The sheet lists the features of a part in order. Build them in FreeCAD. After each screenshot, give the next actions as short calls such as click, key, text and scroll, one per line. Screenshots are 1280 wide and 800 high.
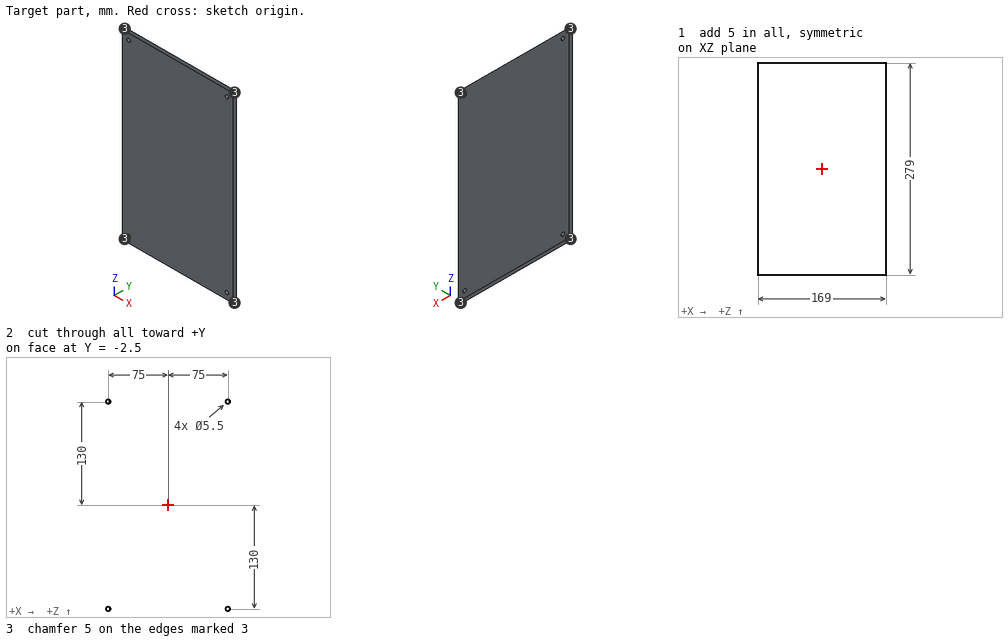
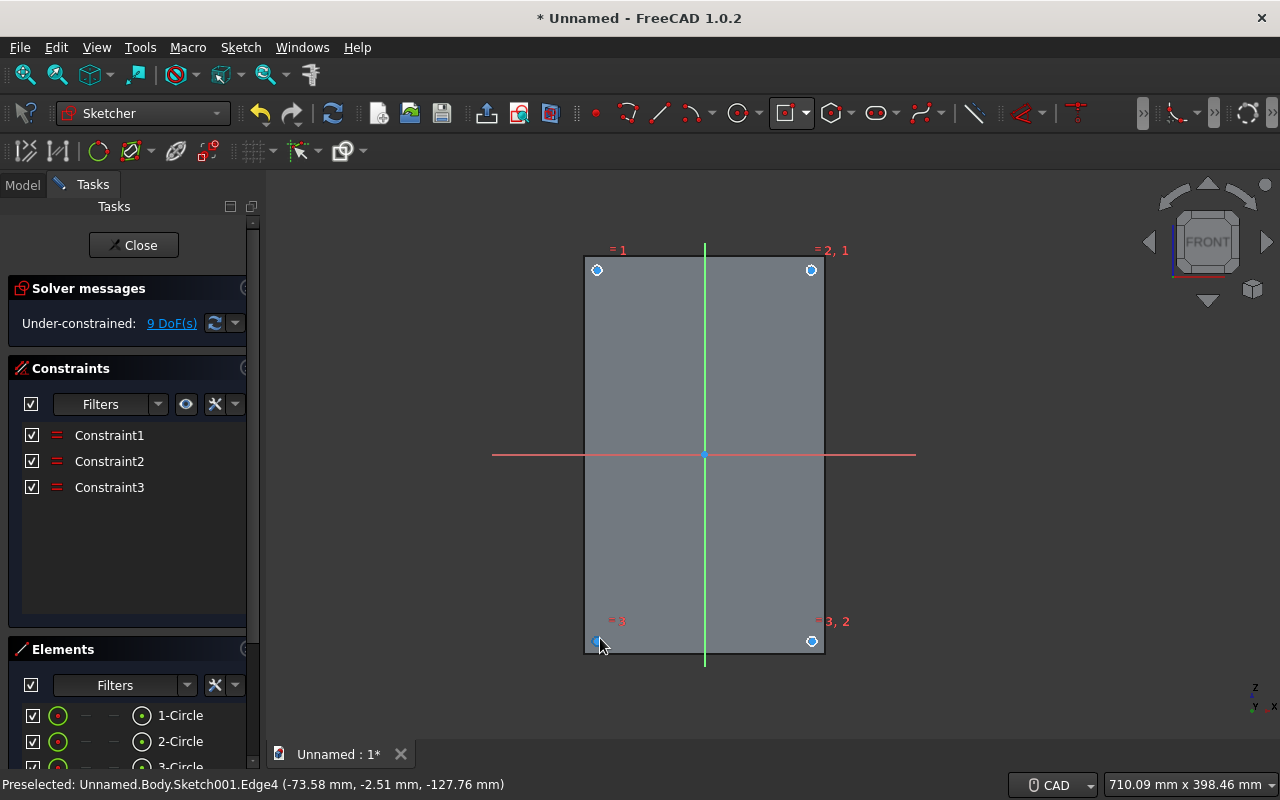
click(597, 270)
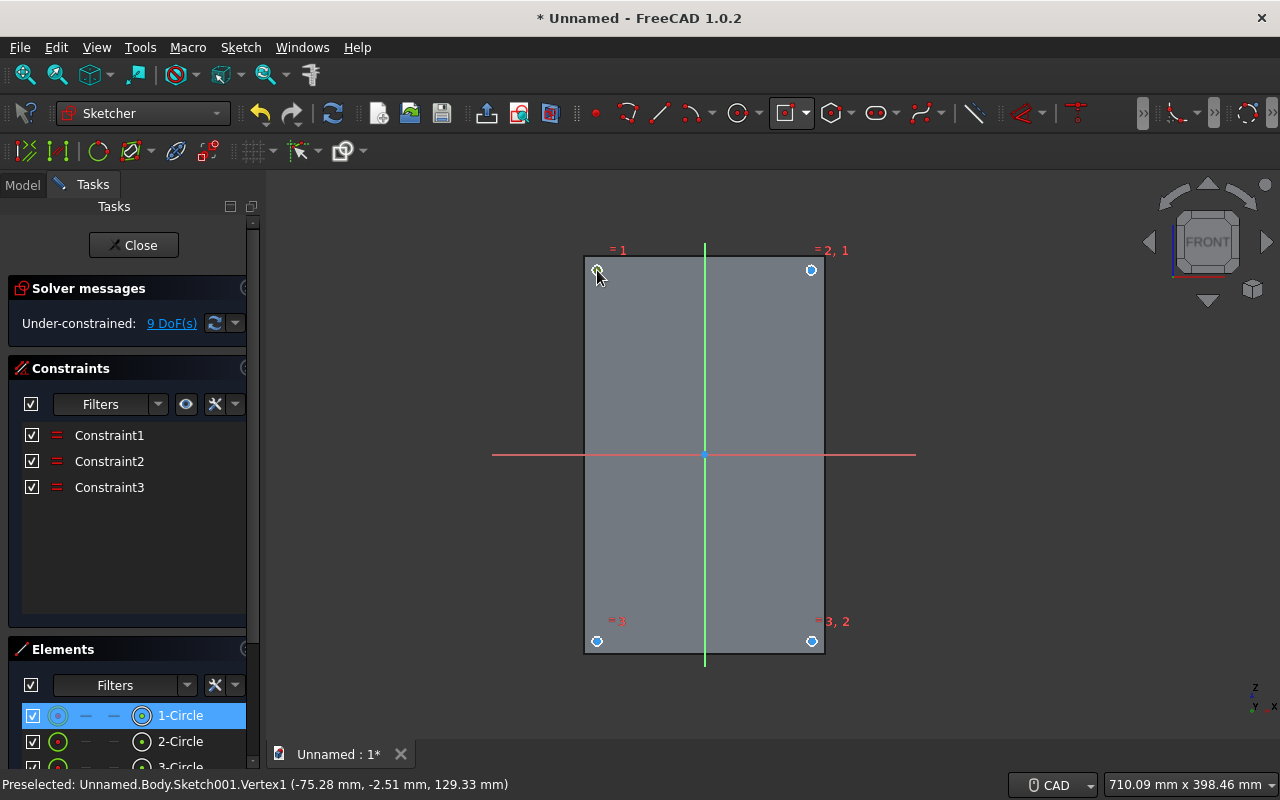
click(811, 270)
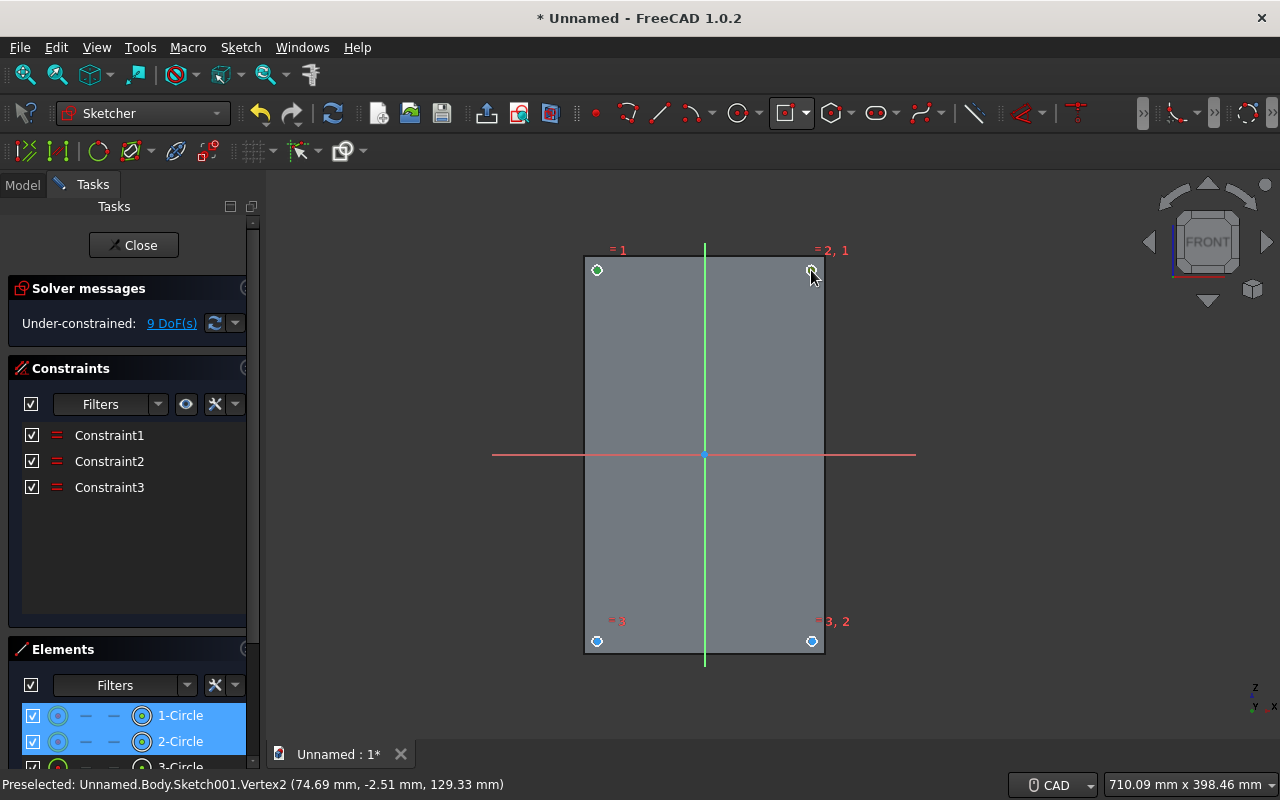
key(h)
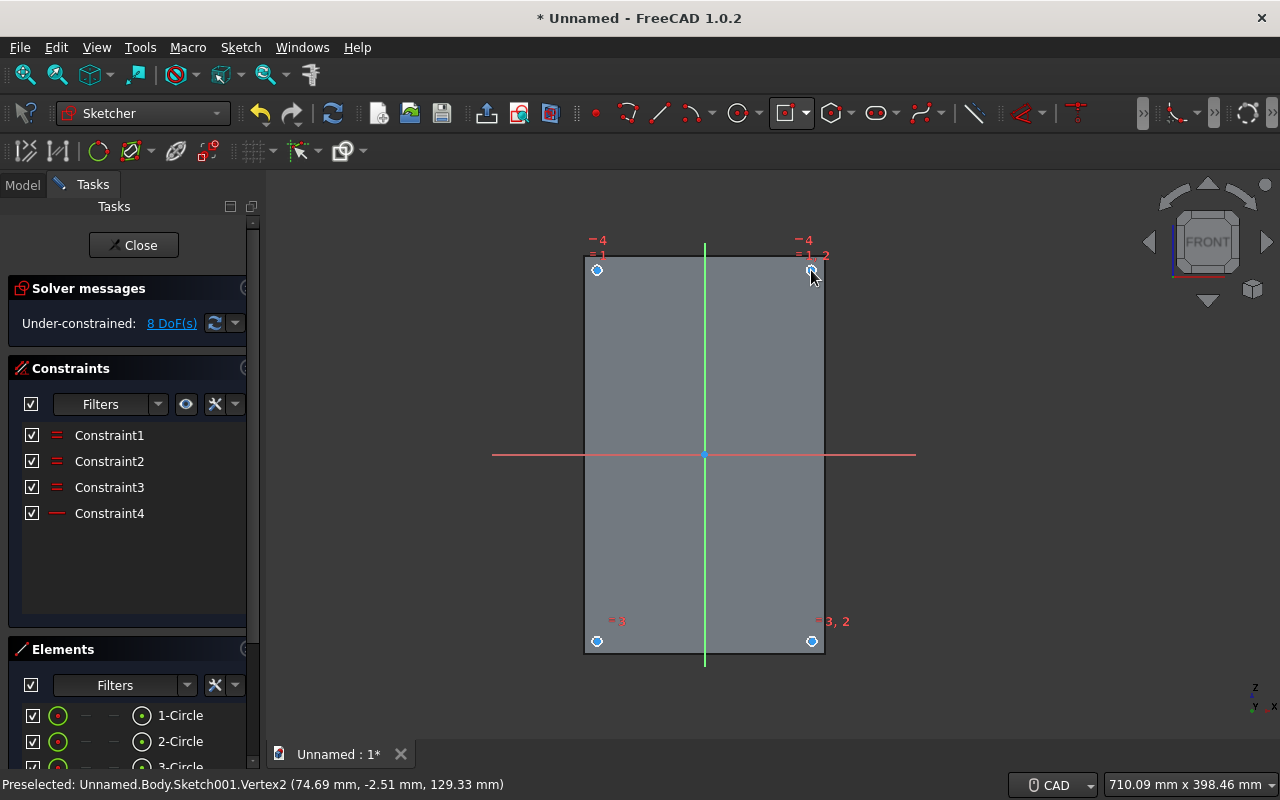
click(811, 270)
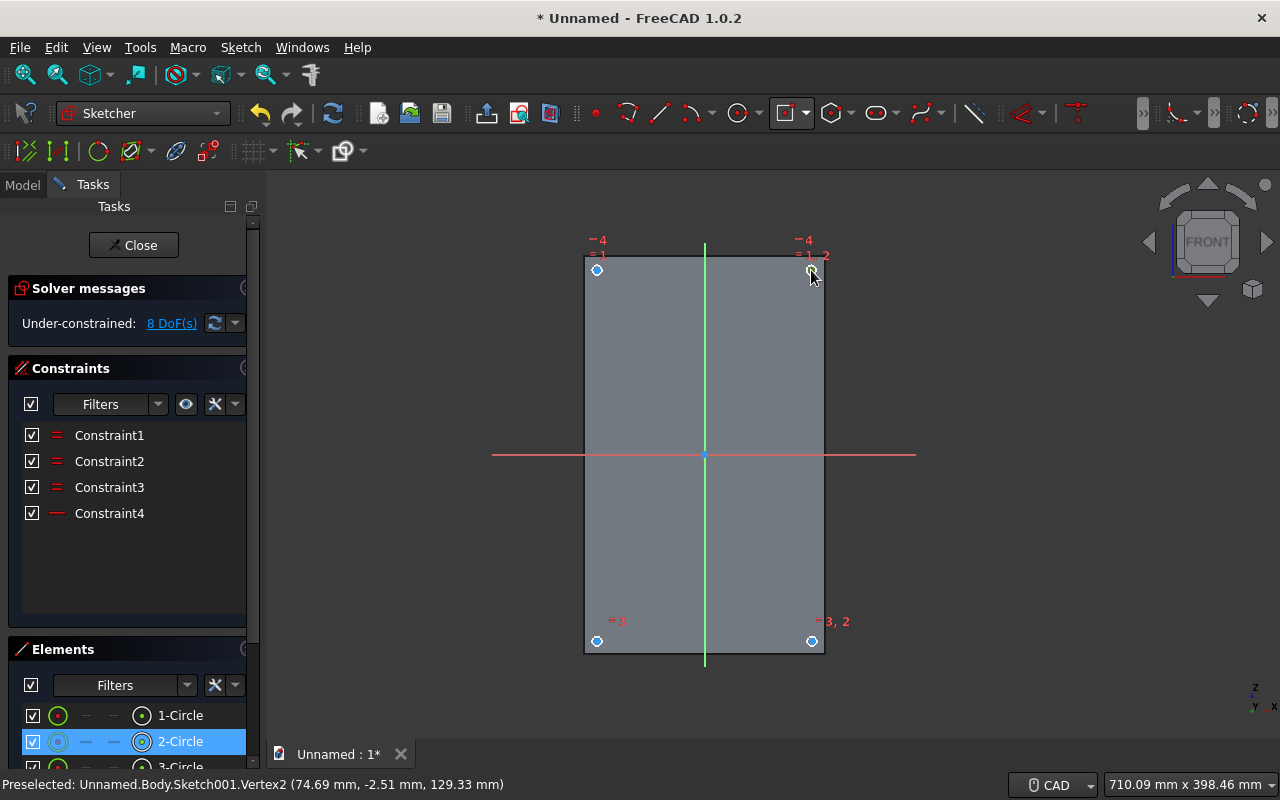
click(812, 641)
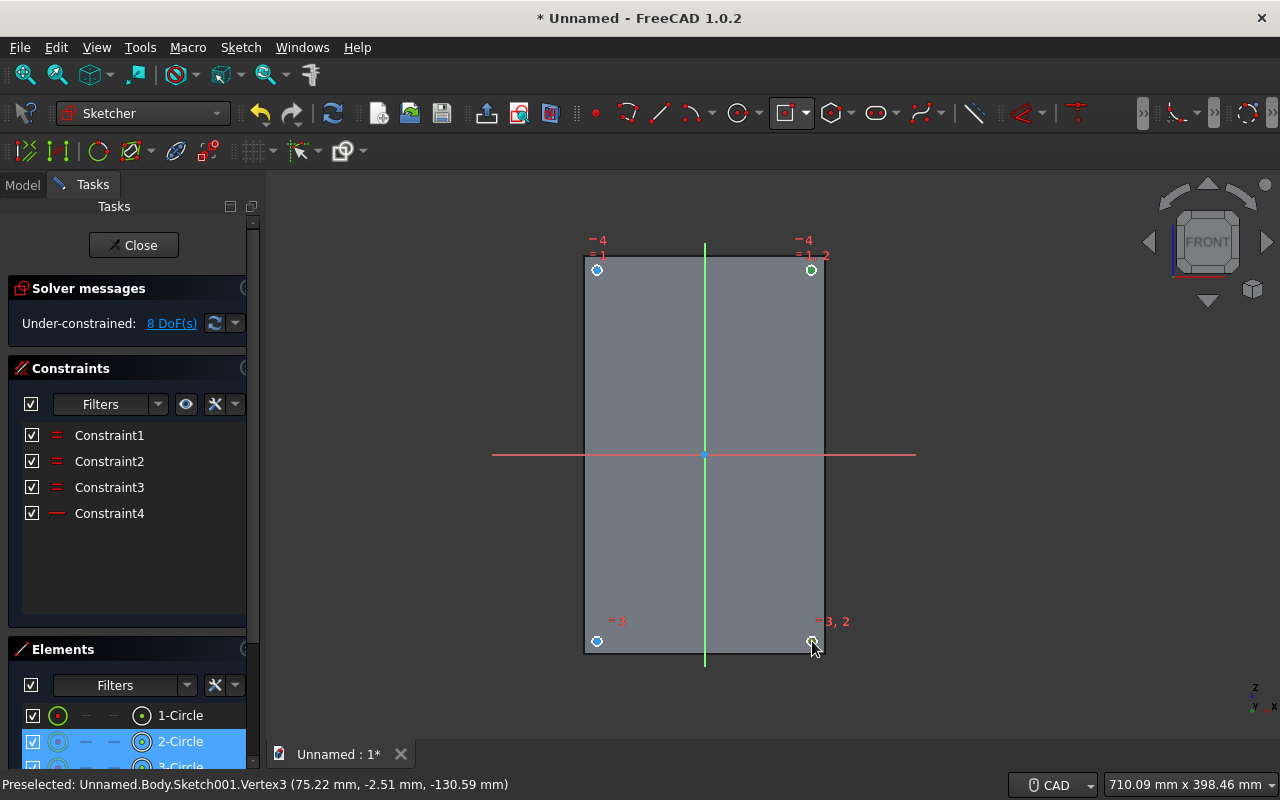
key(v)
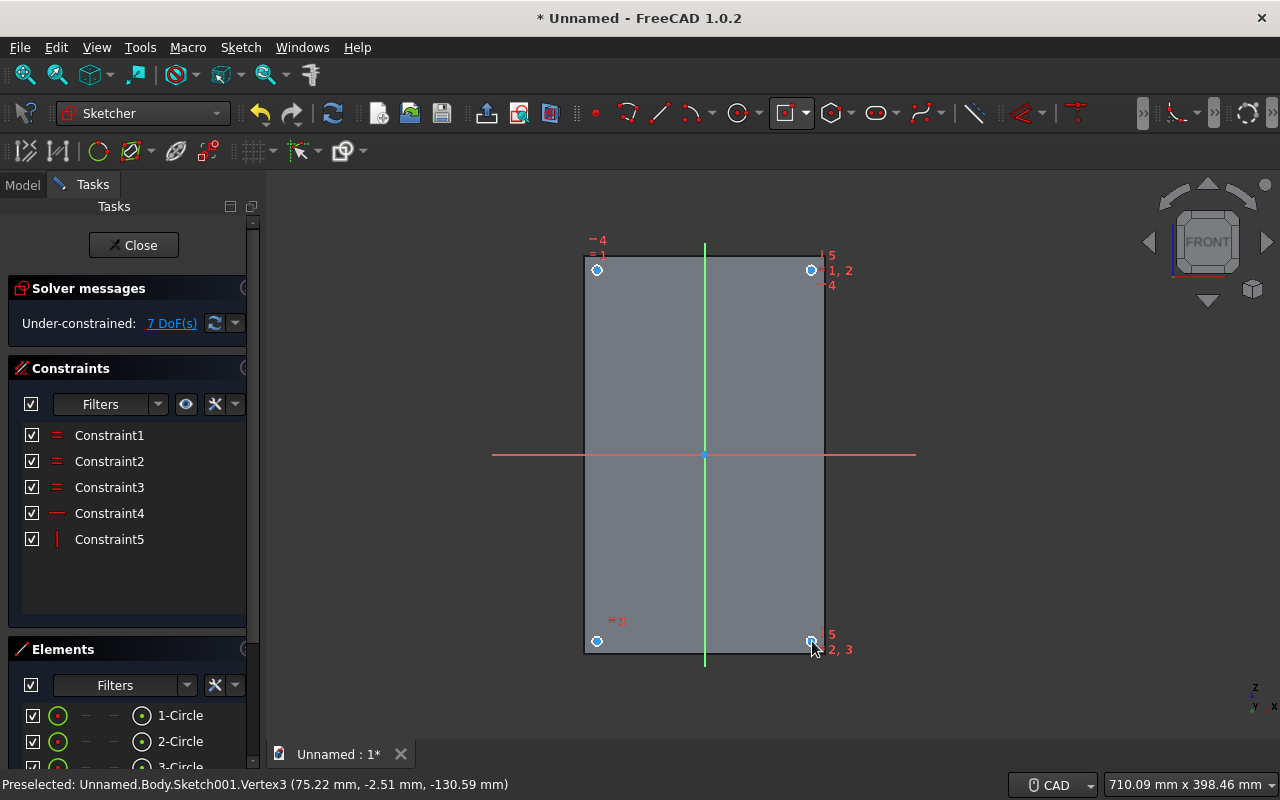
click(597, 270)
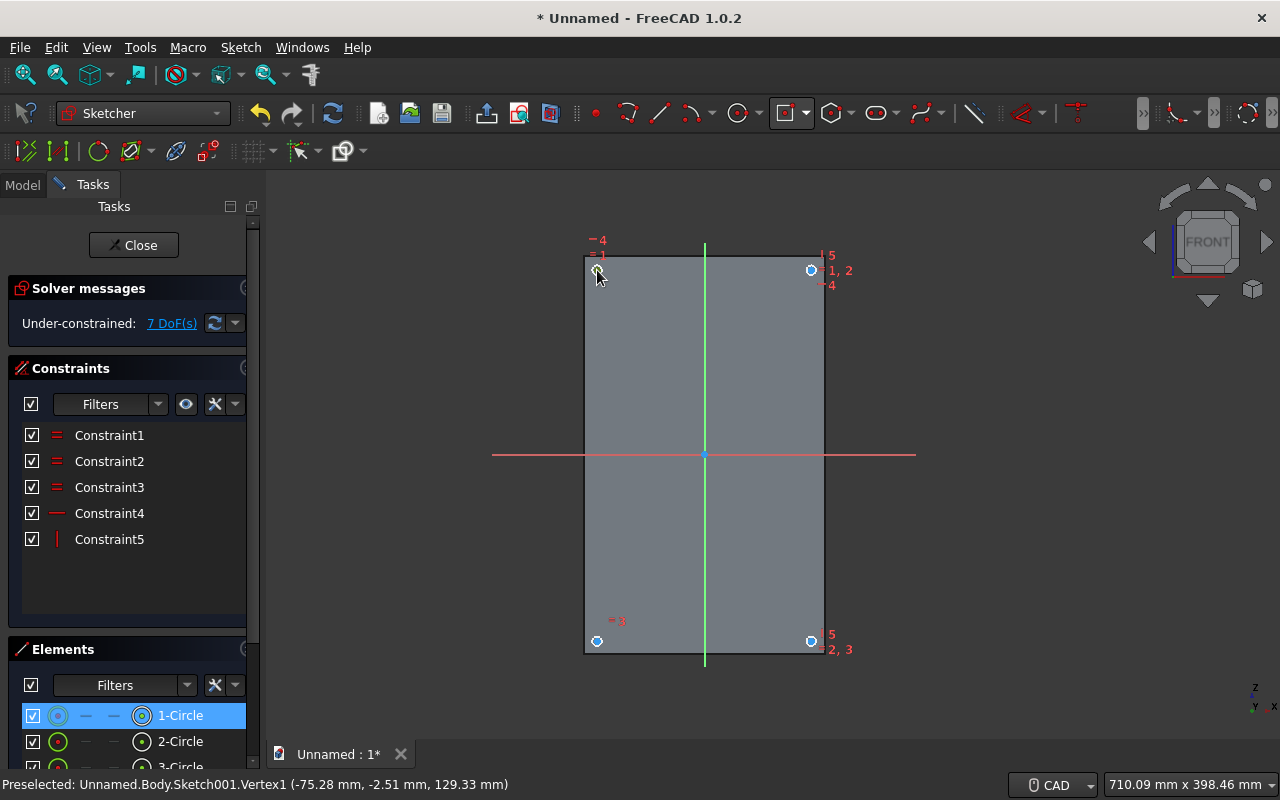
click(597, 641)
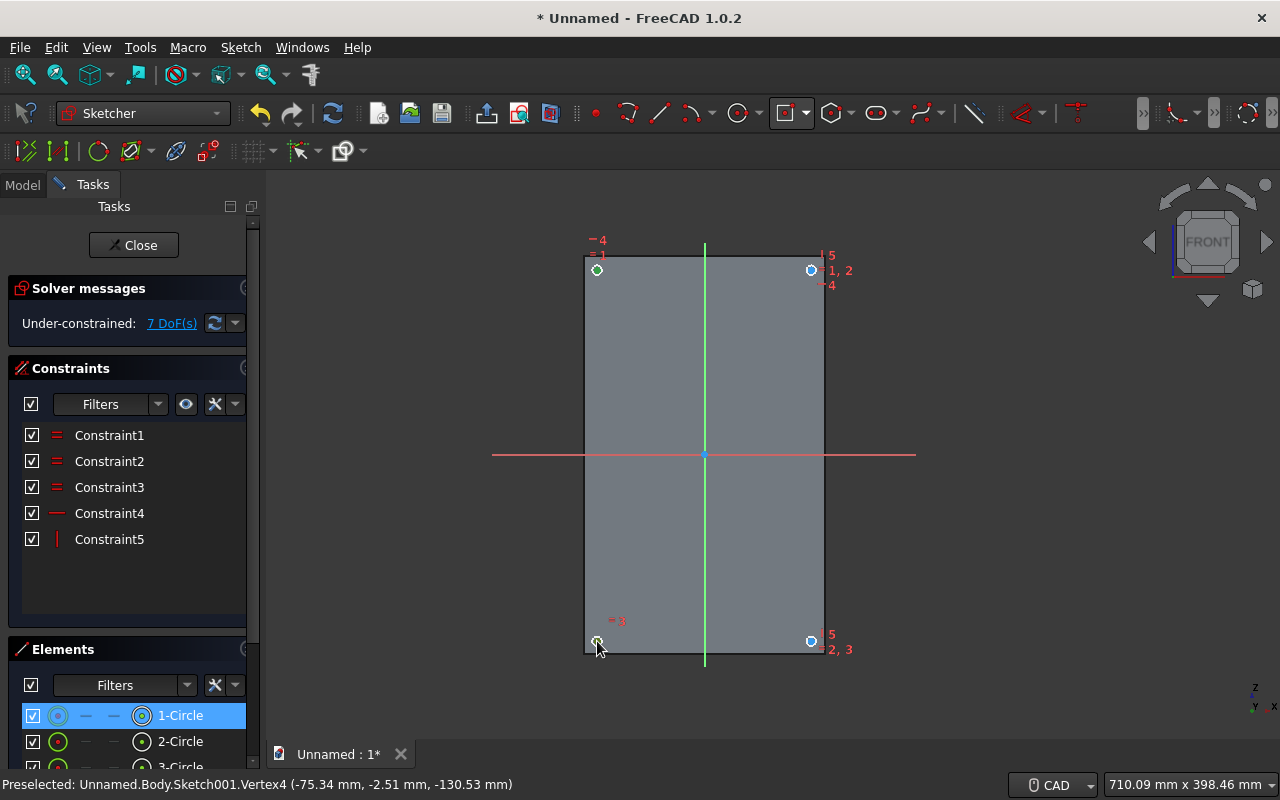
key(v)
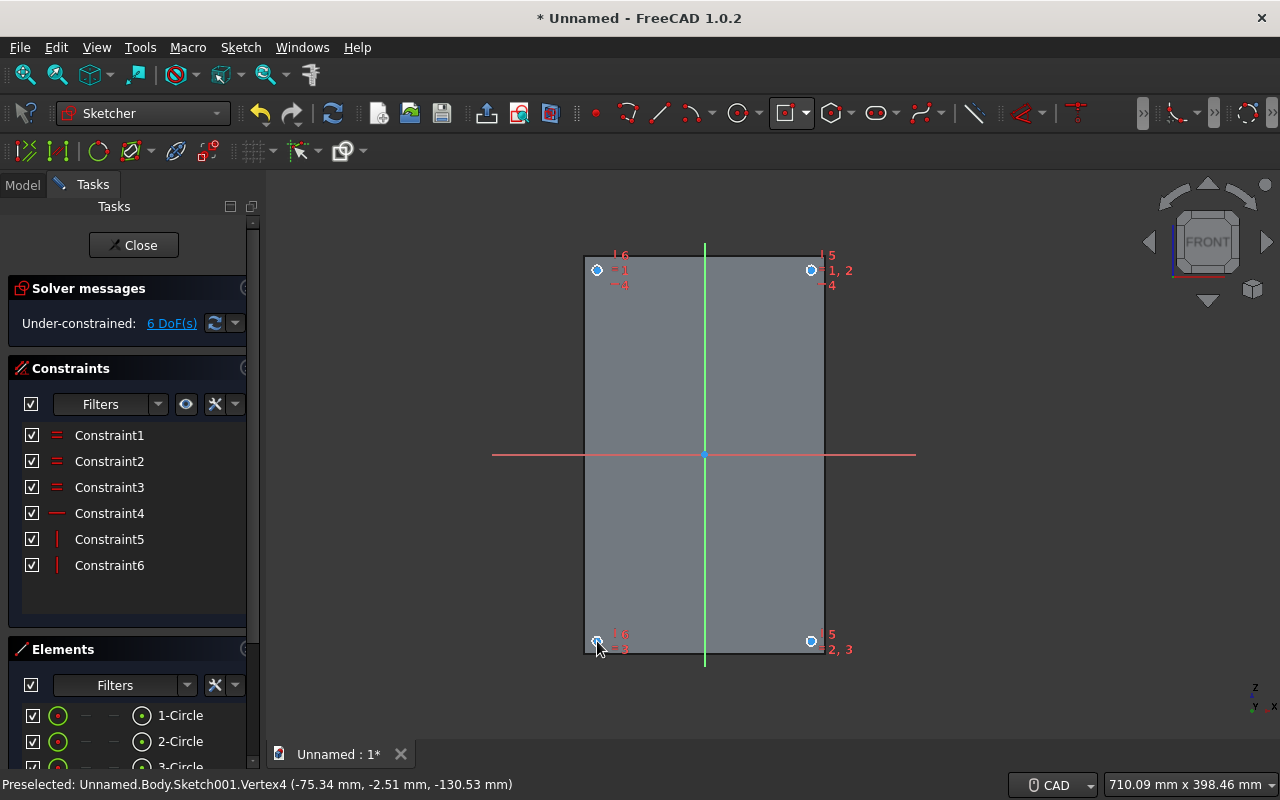
click(811, 641)